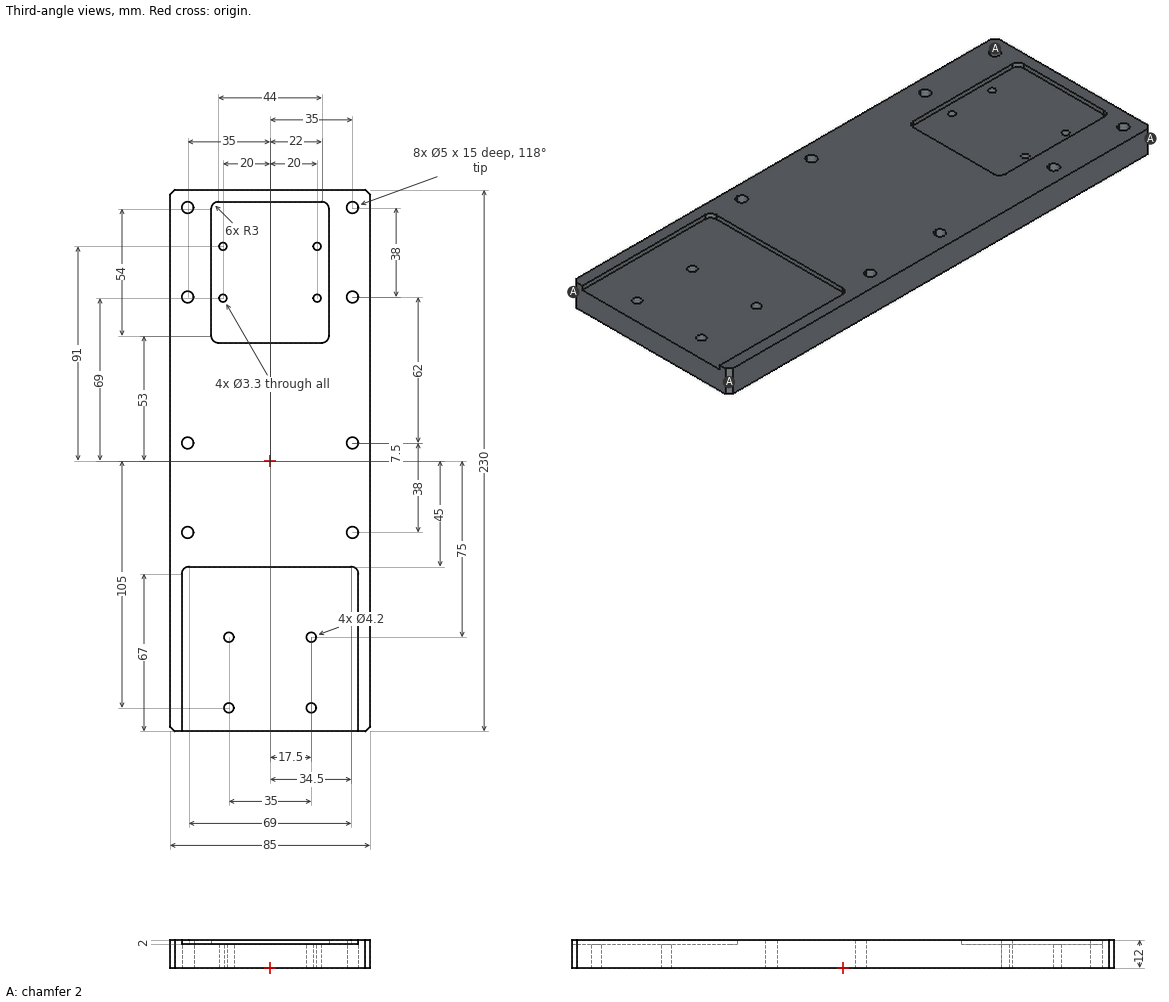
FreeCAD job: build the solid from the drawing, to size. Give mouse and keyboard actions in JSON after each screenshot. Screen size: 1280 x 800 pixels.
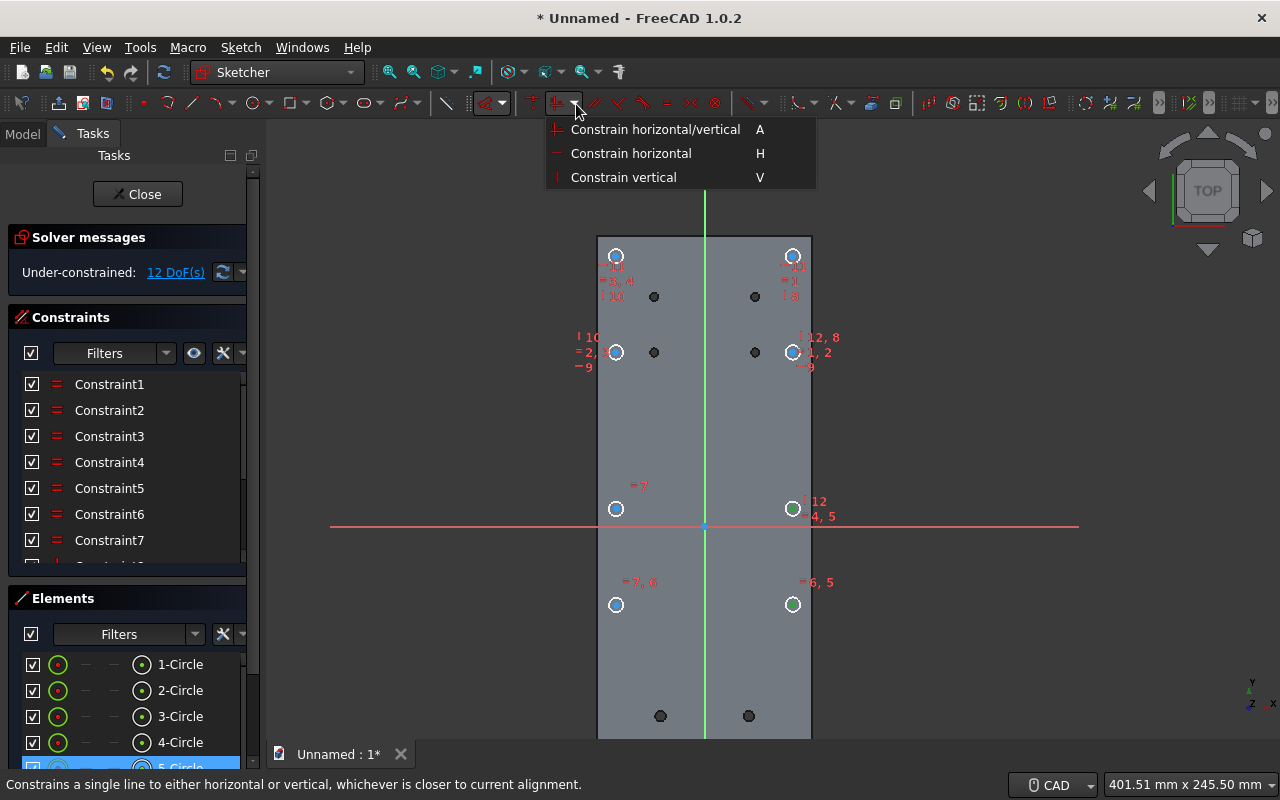
{"action": "left_click", "coordinate": [681, 177]}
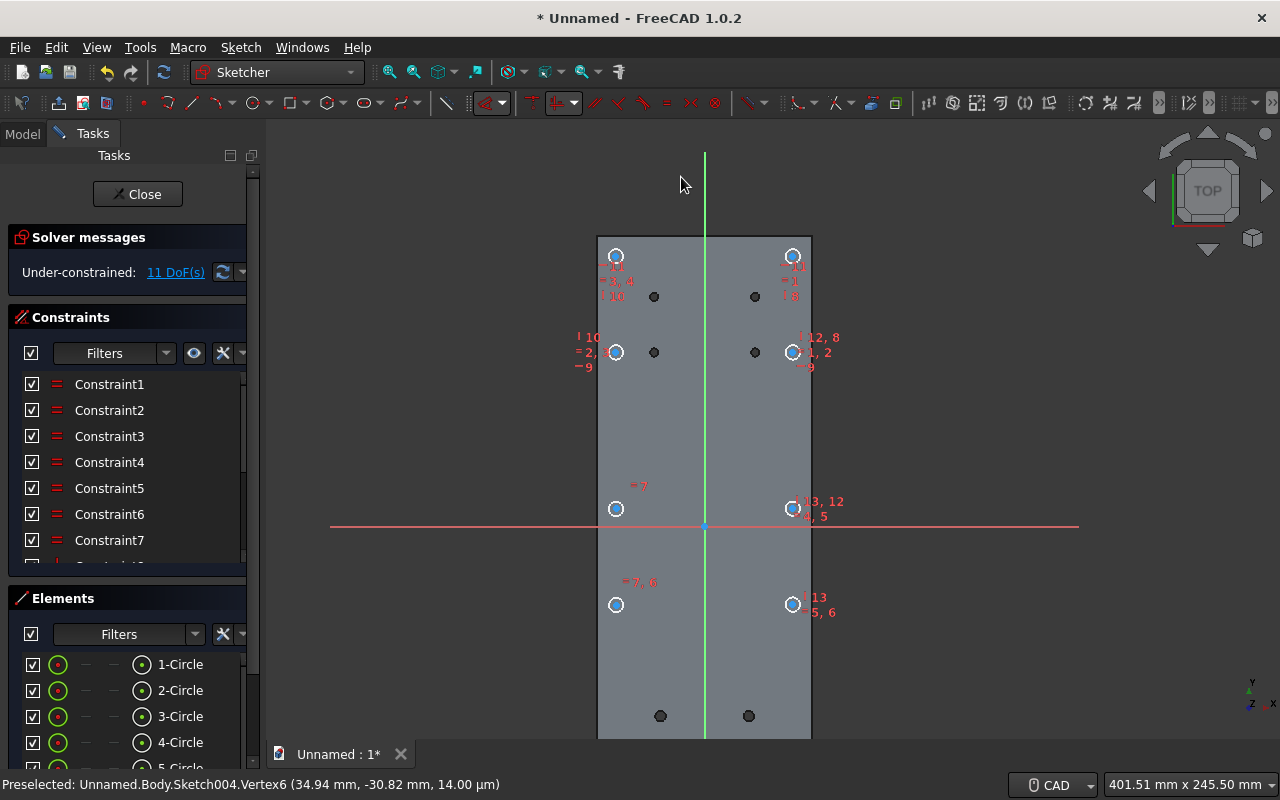
{"action": "left_click", "coordinate": [616, 352]}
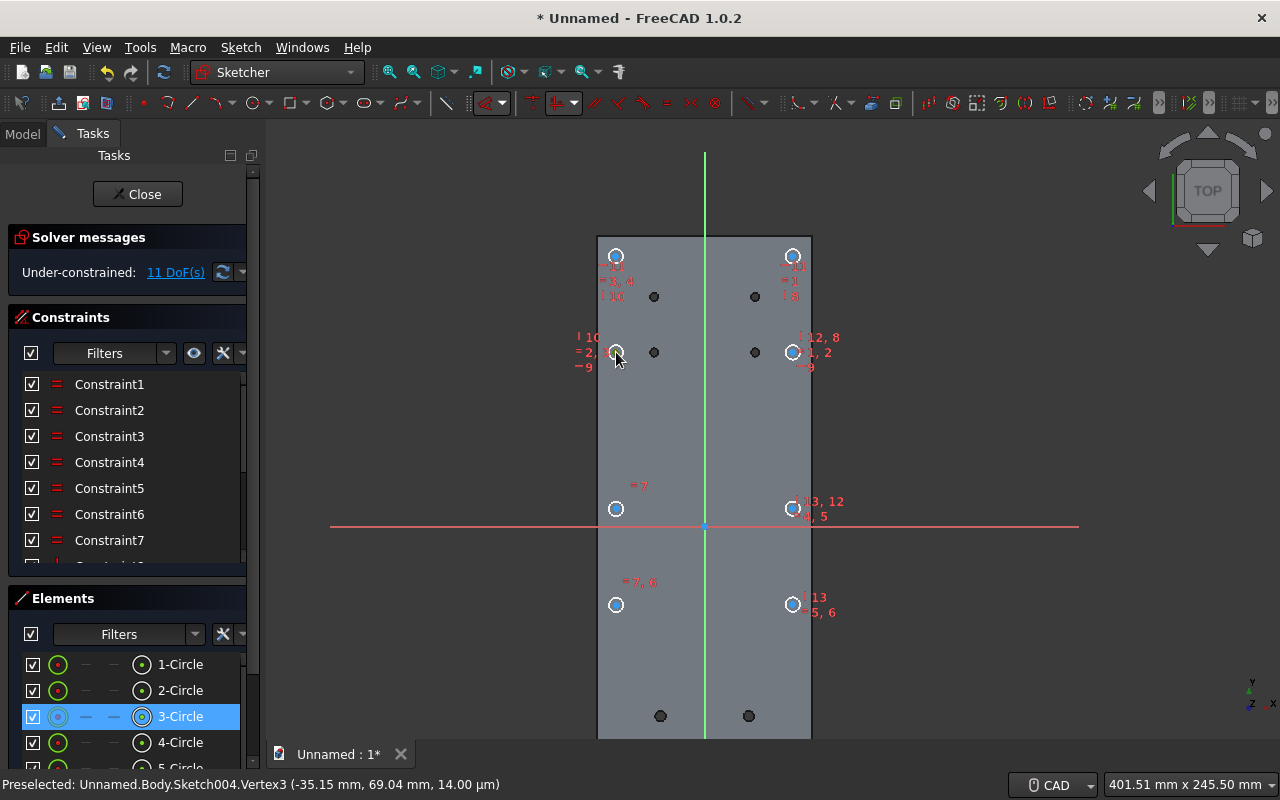
{"action": "left_click", "coordinate": [616, 605]}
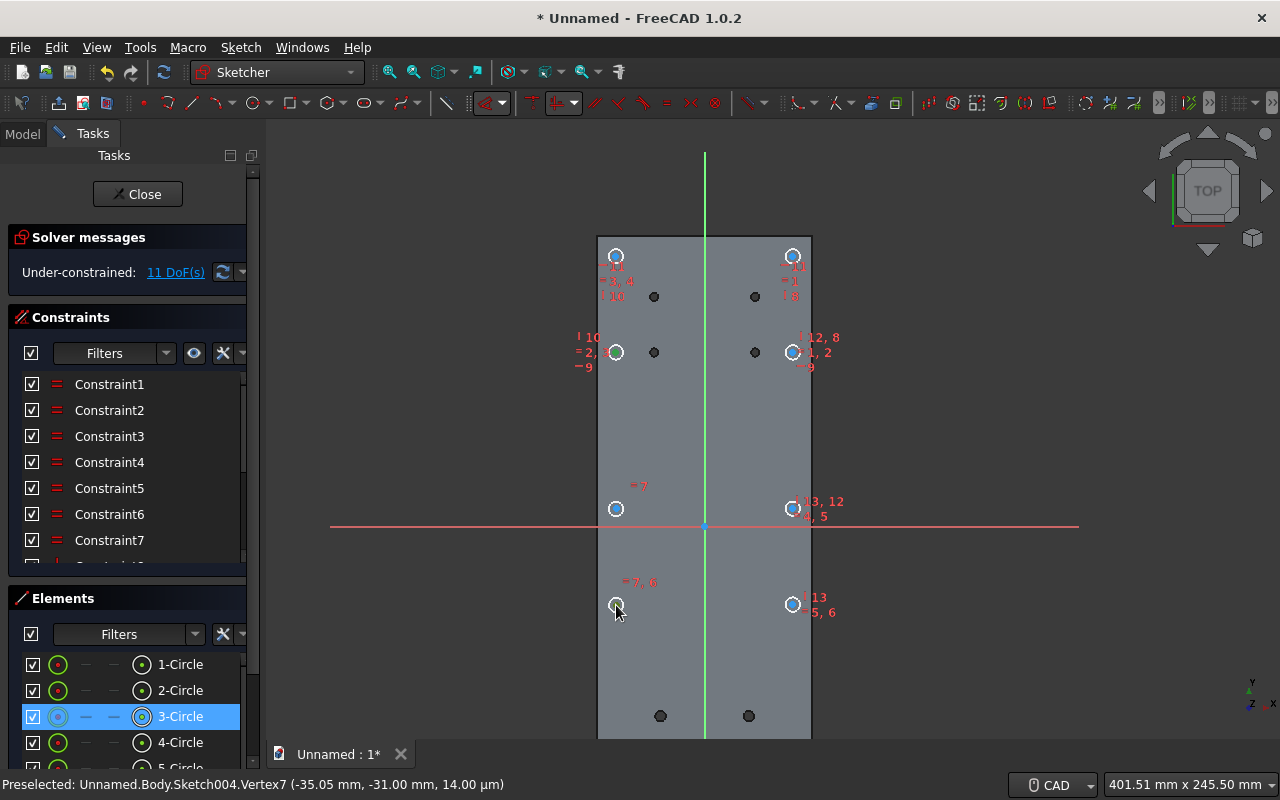
{"action": "key", "text": "v"}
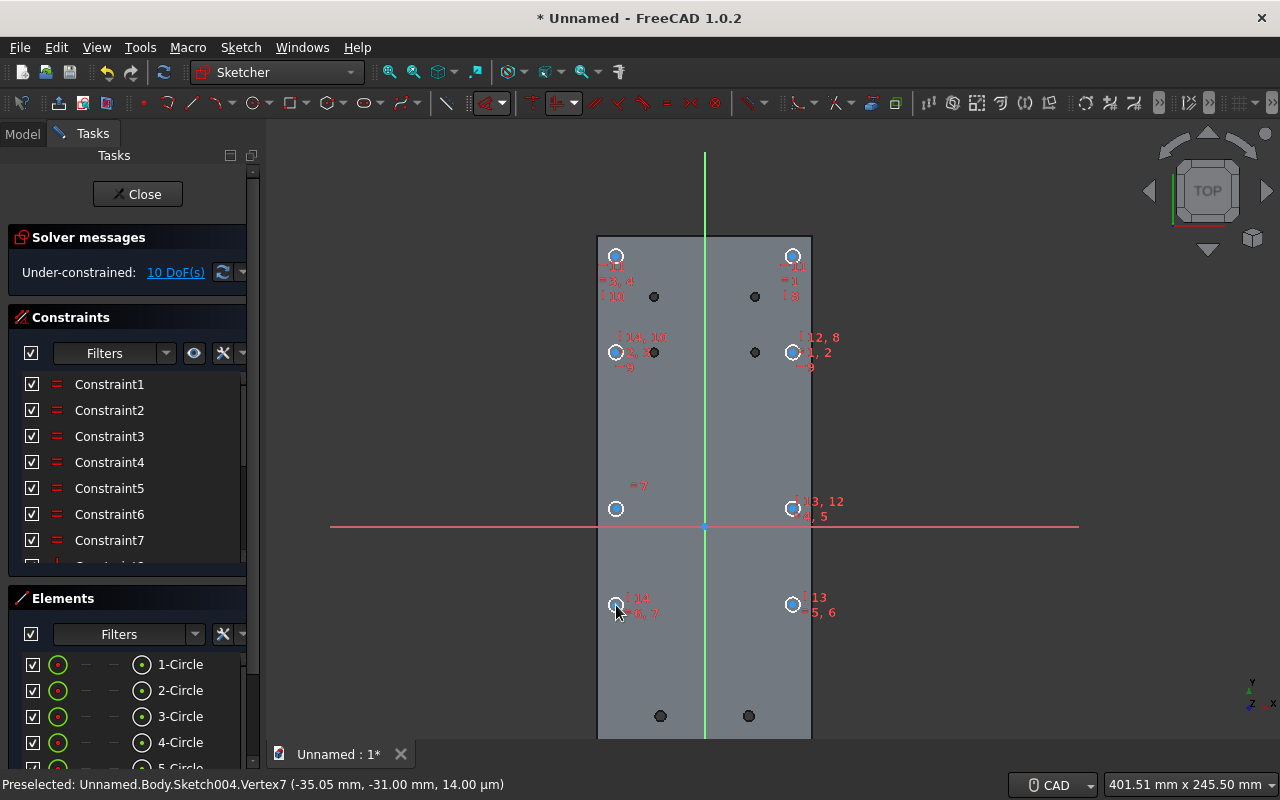
{"action": "left_click", "coordinate": [793, 605]}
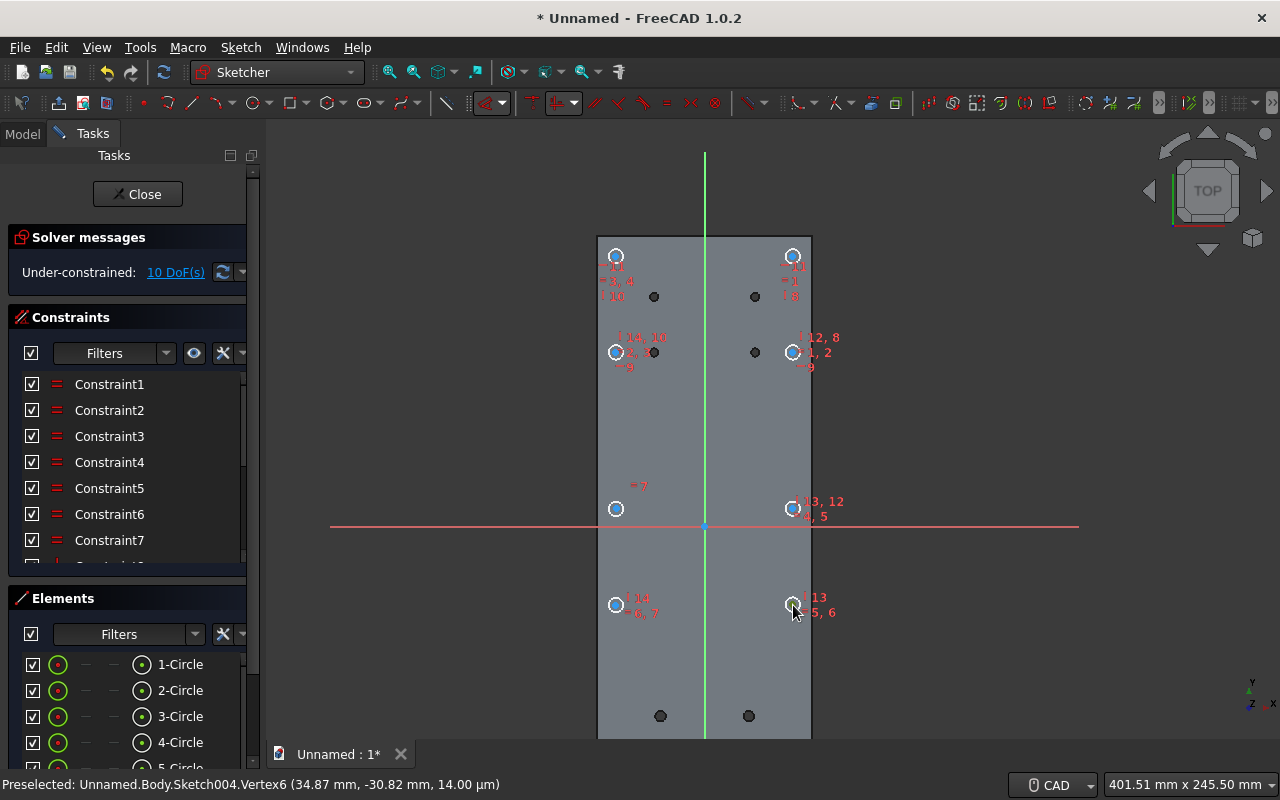
{"action": "left_click", "coordinate": [616, 605]}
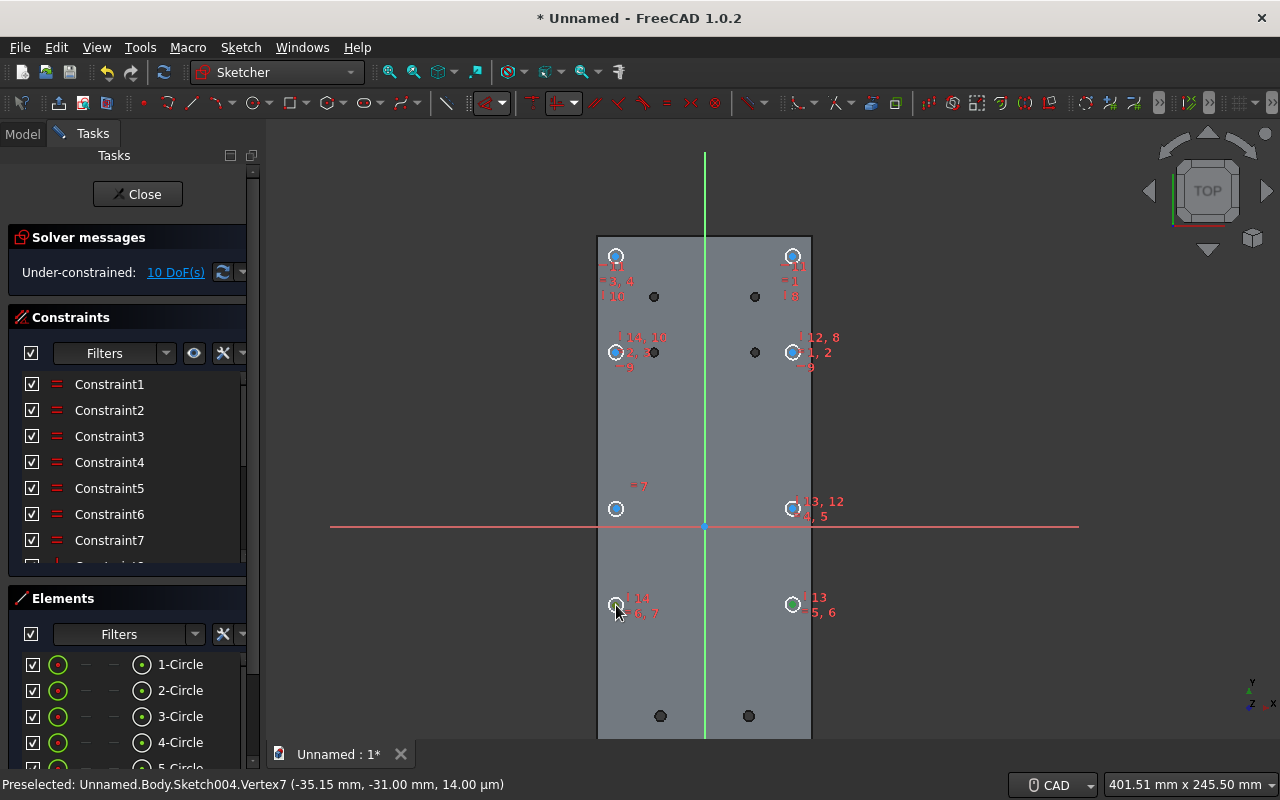
{"action": "left_click", "coordinate": [576, 104]}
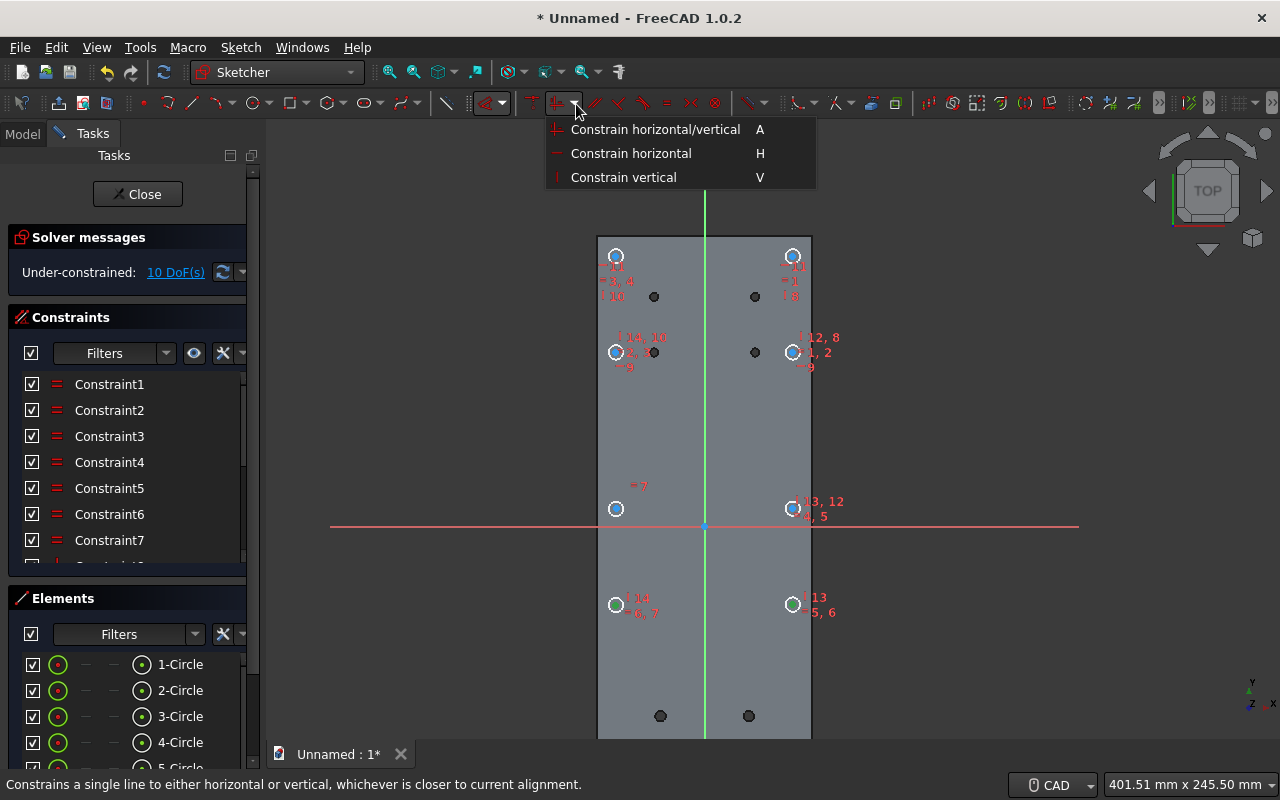
{"action": "left_click", "coordinate": [681, 153]}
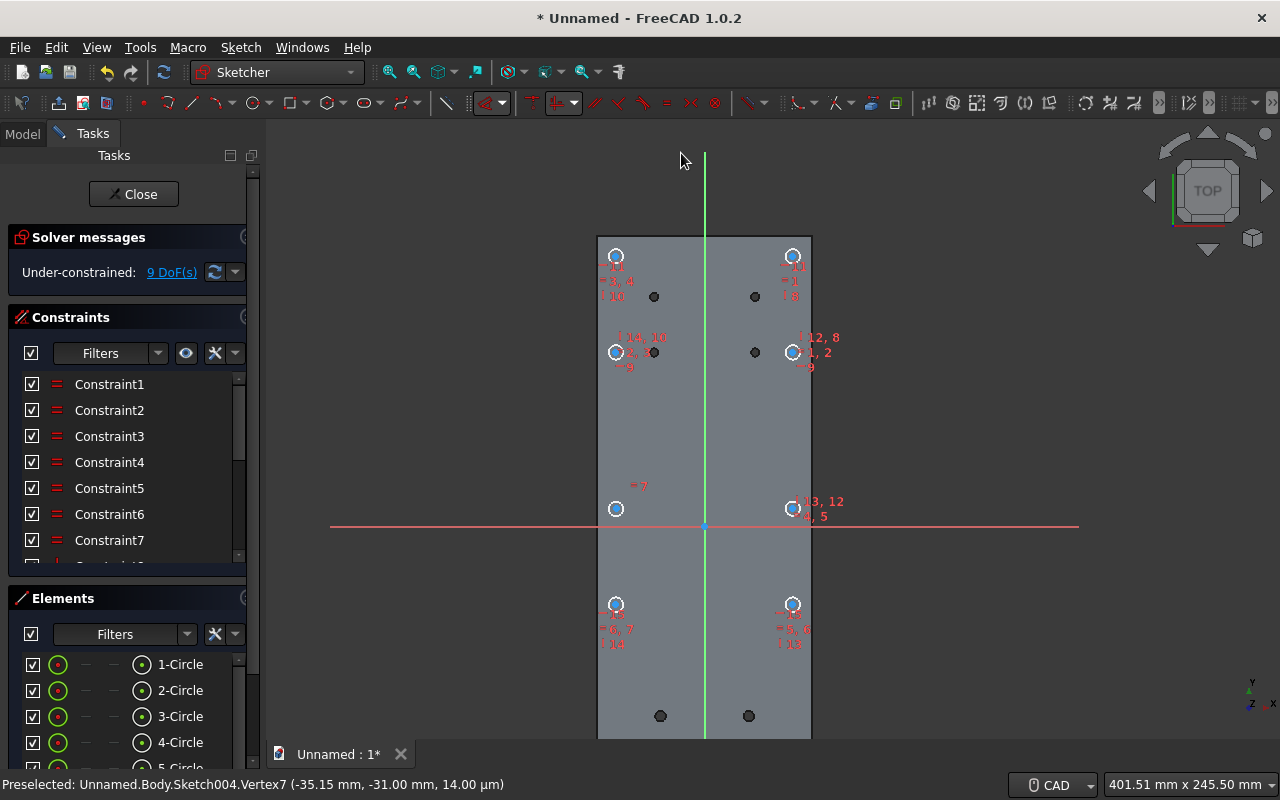
{"action": "left_click", "coordinate": [616, 605]}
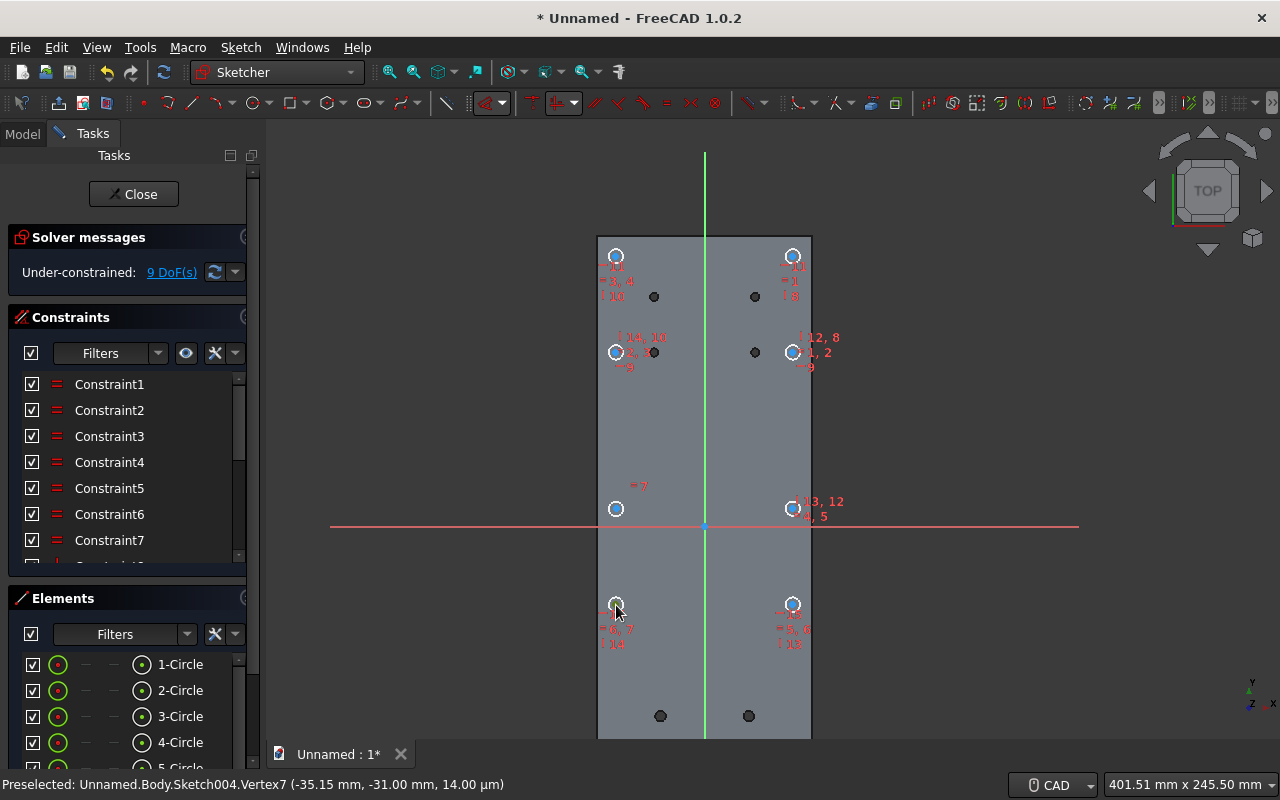
{"action": "left_click", "coordinate": [616, 509]}